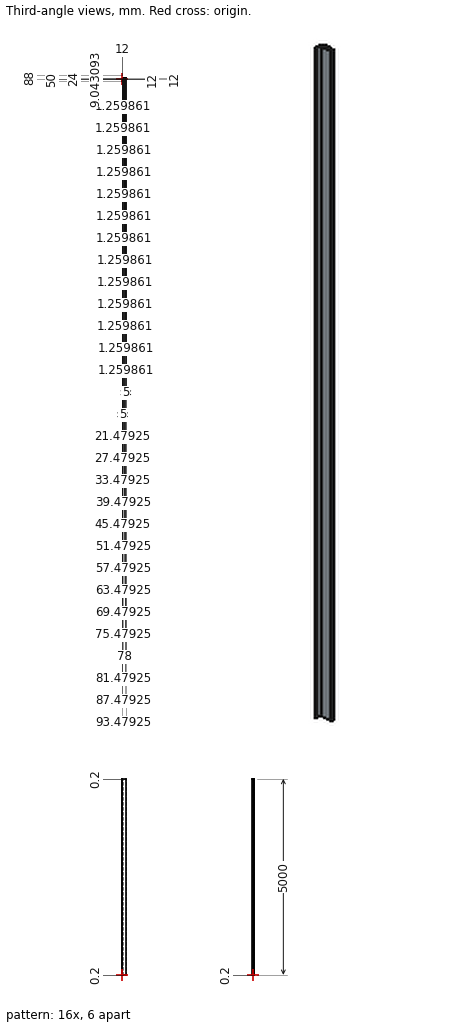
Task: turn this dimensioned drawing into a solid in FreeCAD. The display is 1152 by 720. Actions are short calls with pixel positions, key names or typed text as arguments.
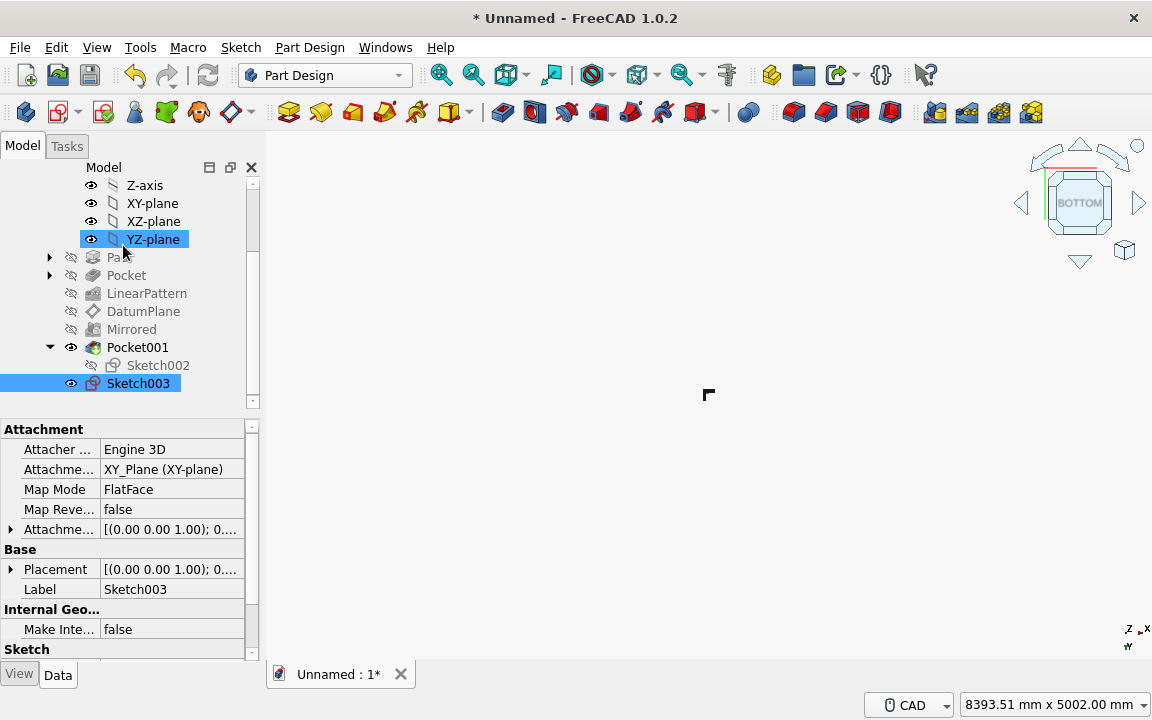
click(504, 112)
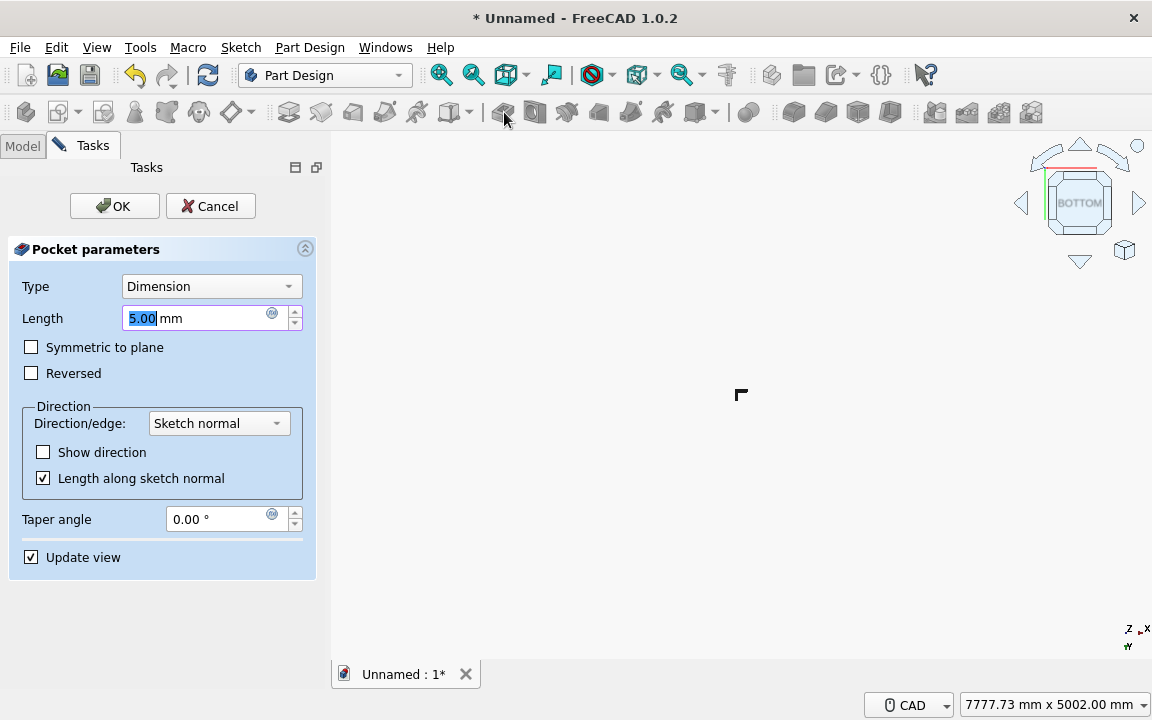
text(0.2)
key(Tab)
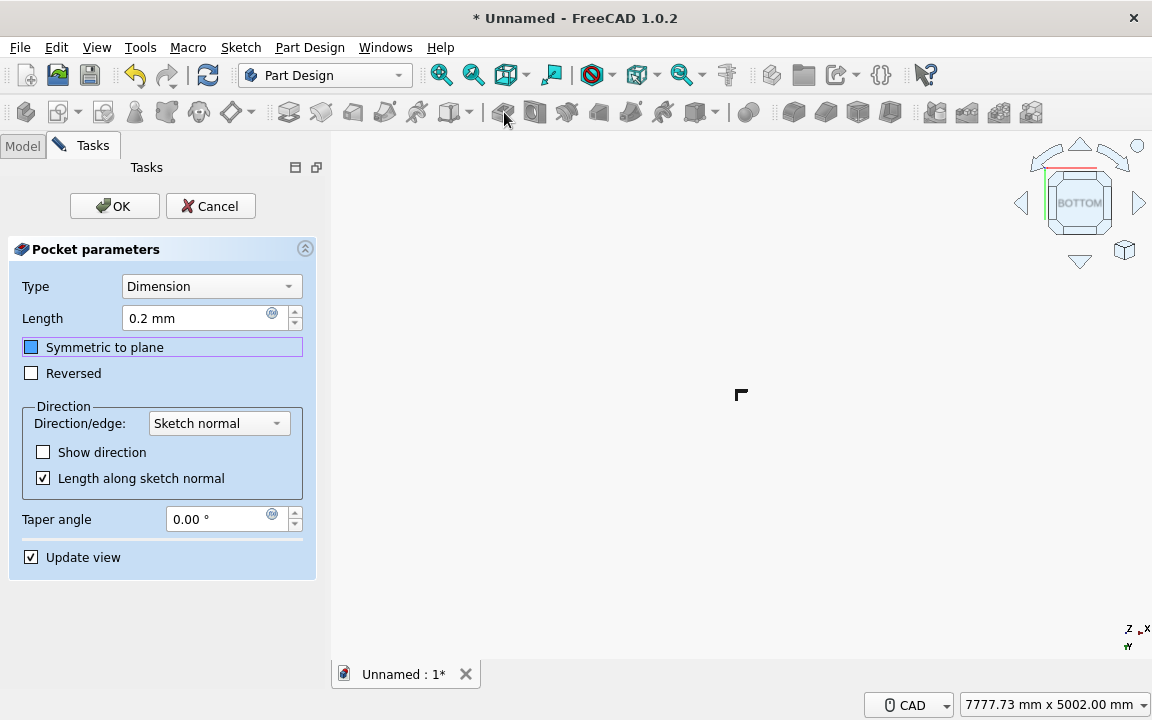
click(30, 373)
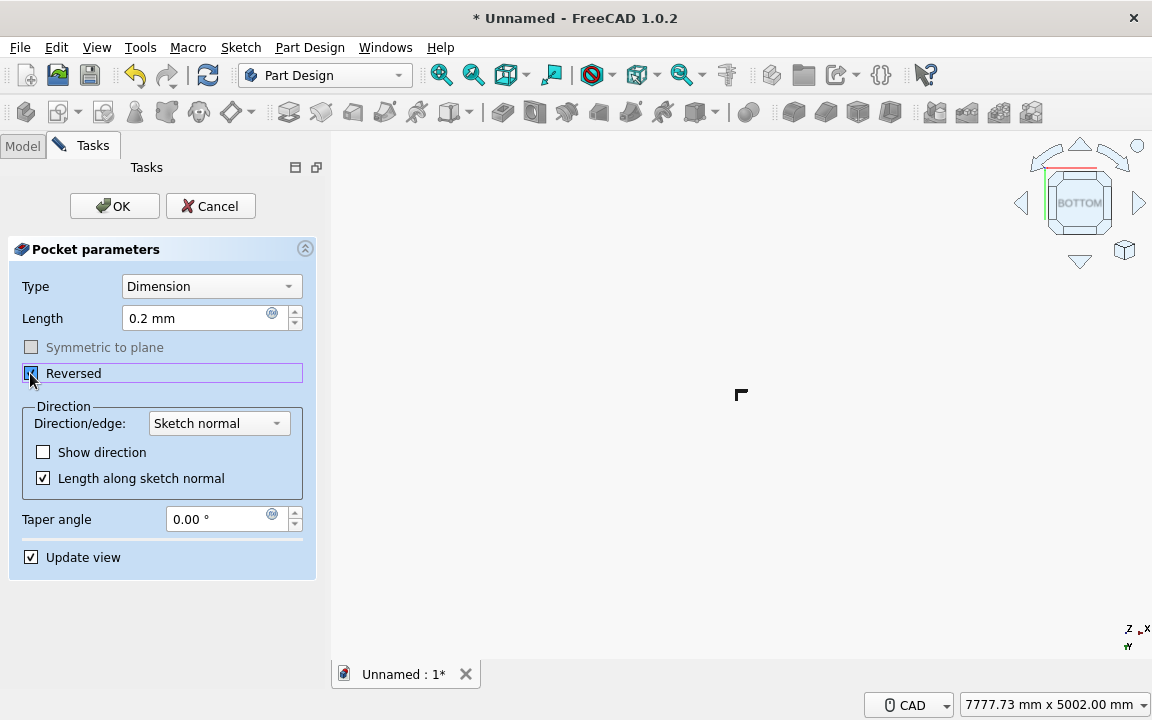
click(115, 206)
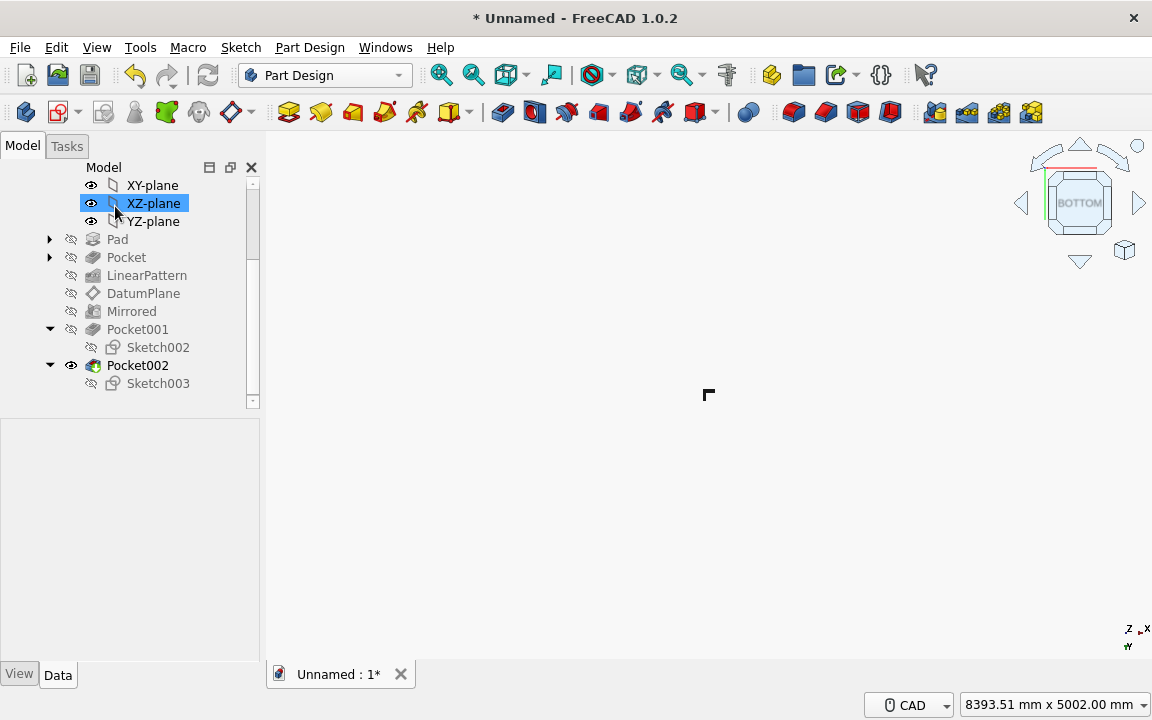
click(442, 76)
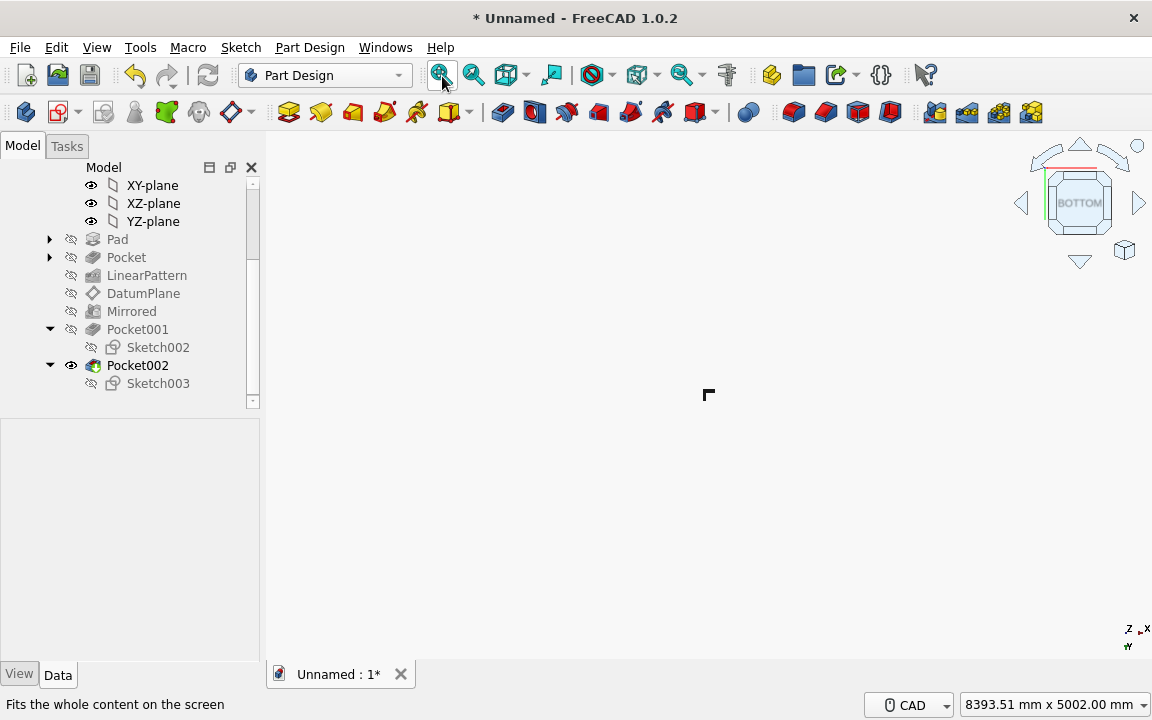
click(58, 112)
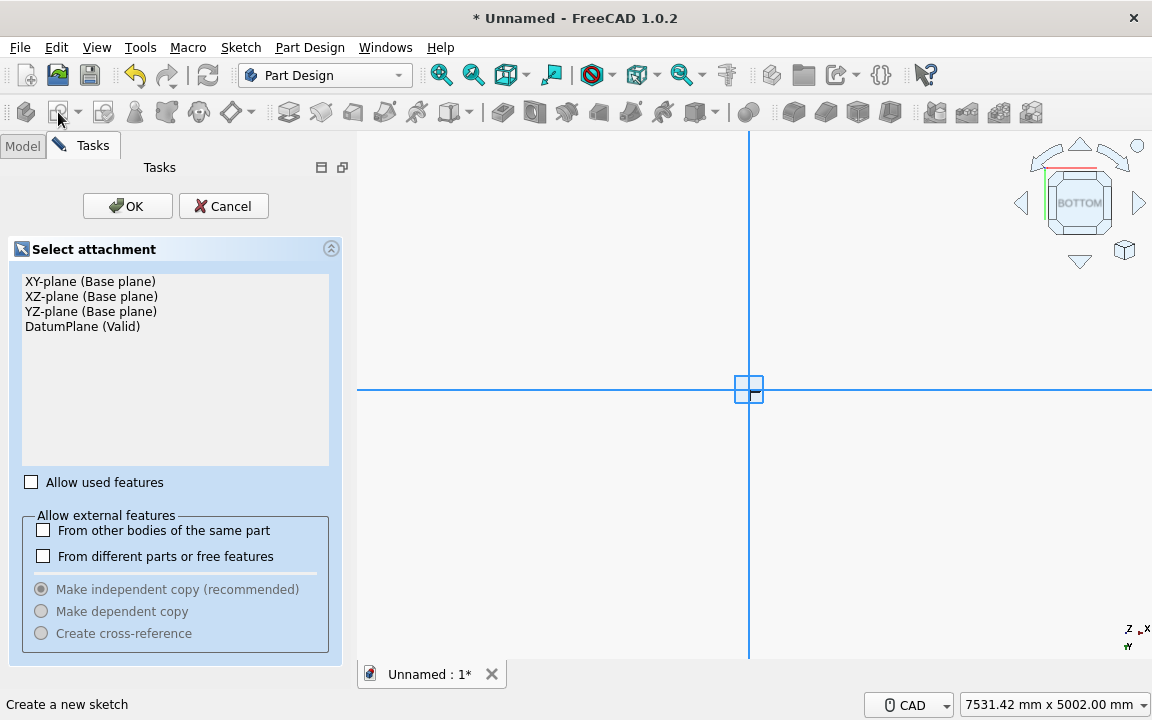
click(82, 282)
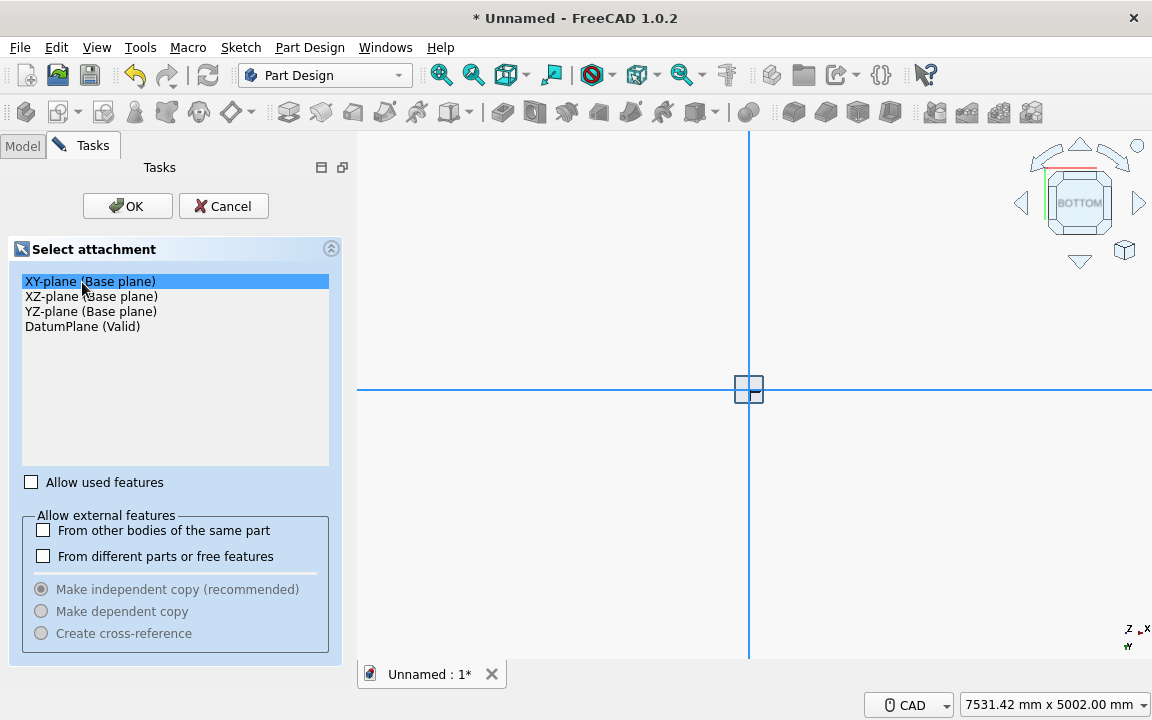
click(128, 206)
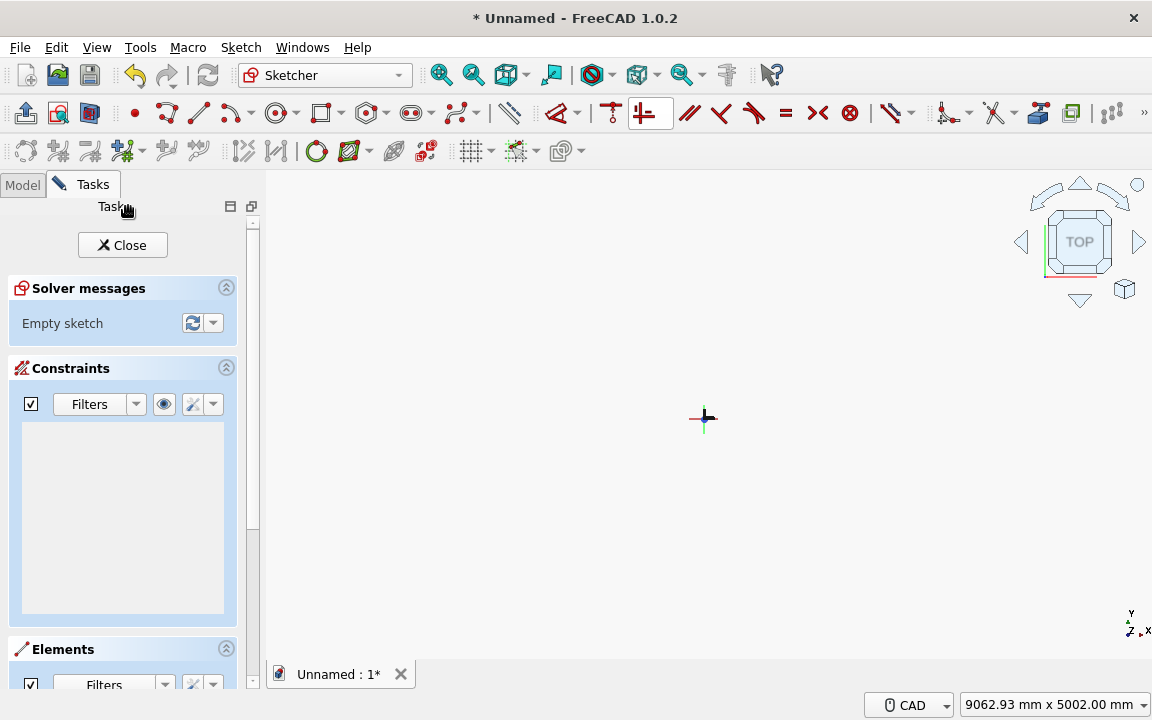
click(90, 114)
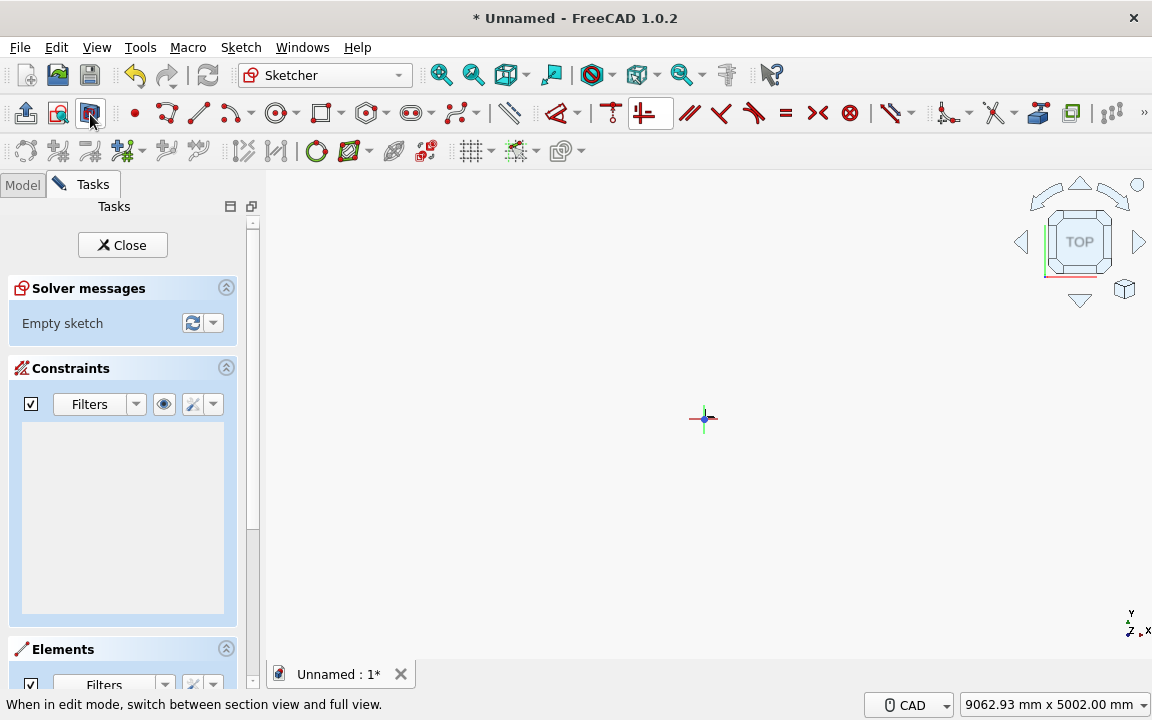
scroll(712, 418, up, 15)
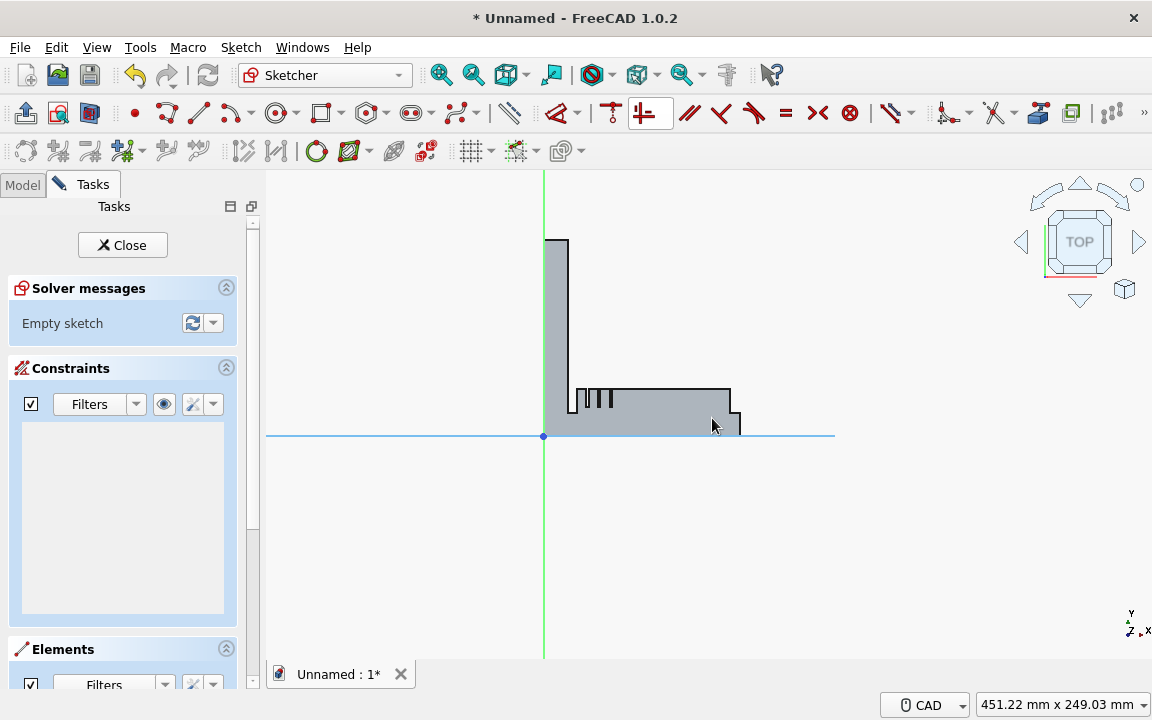
scroll(622, 397, up, 14)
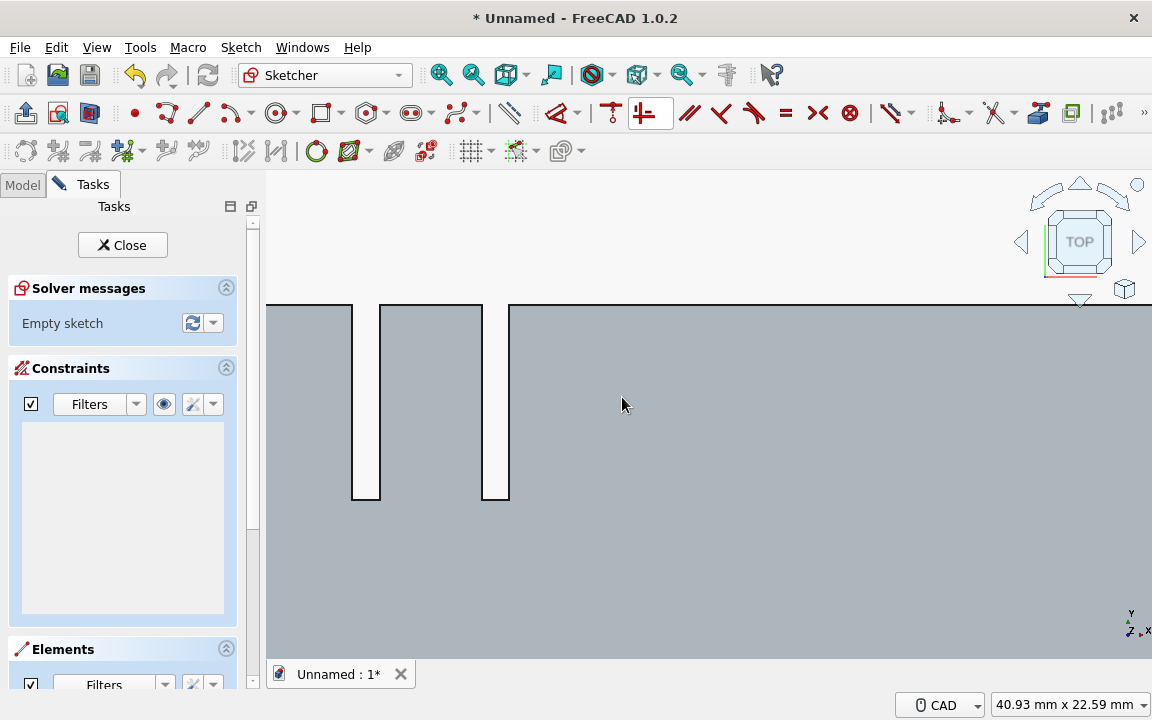
click(322, 114)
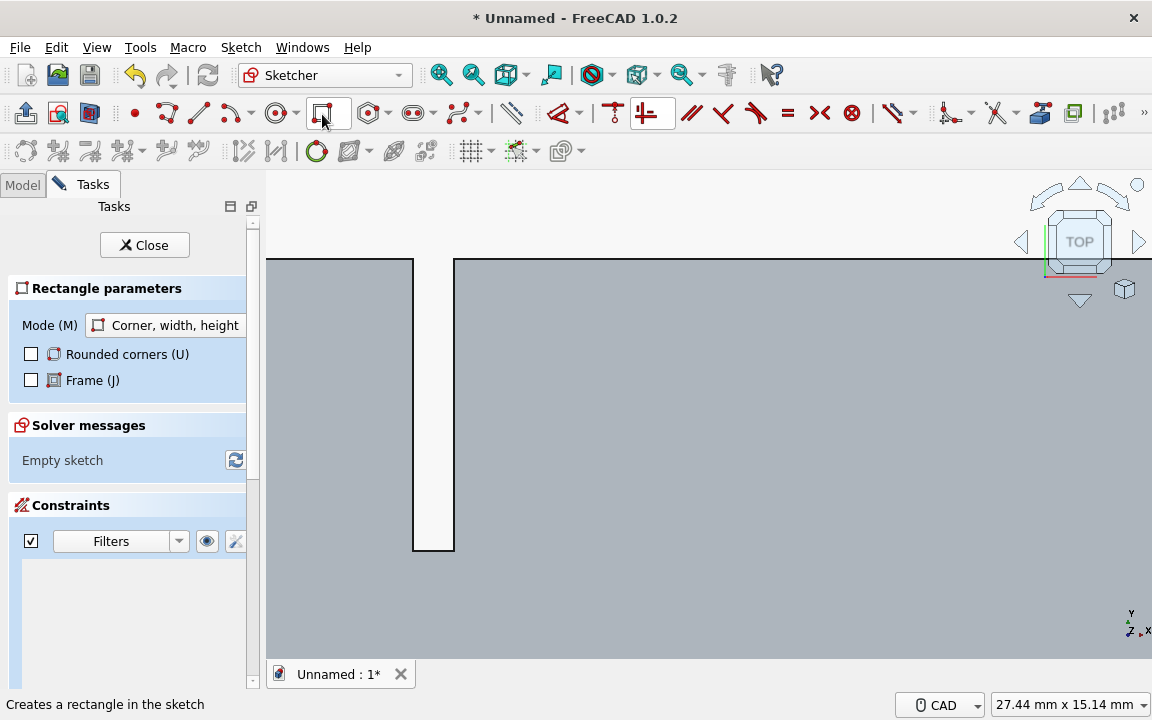
click(607, 259)
click(648, 551)
key(Escape)